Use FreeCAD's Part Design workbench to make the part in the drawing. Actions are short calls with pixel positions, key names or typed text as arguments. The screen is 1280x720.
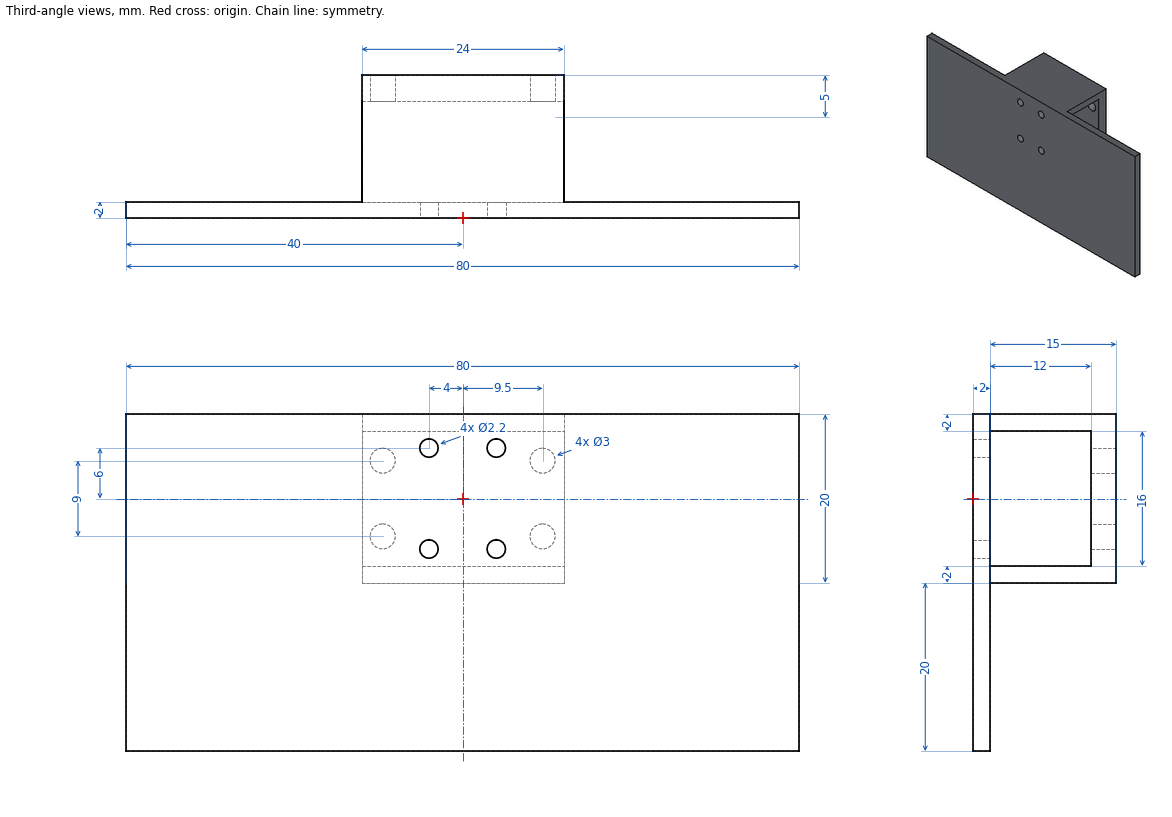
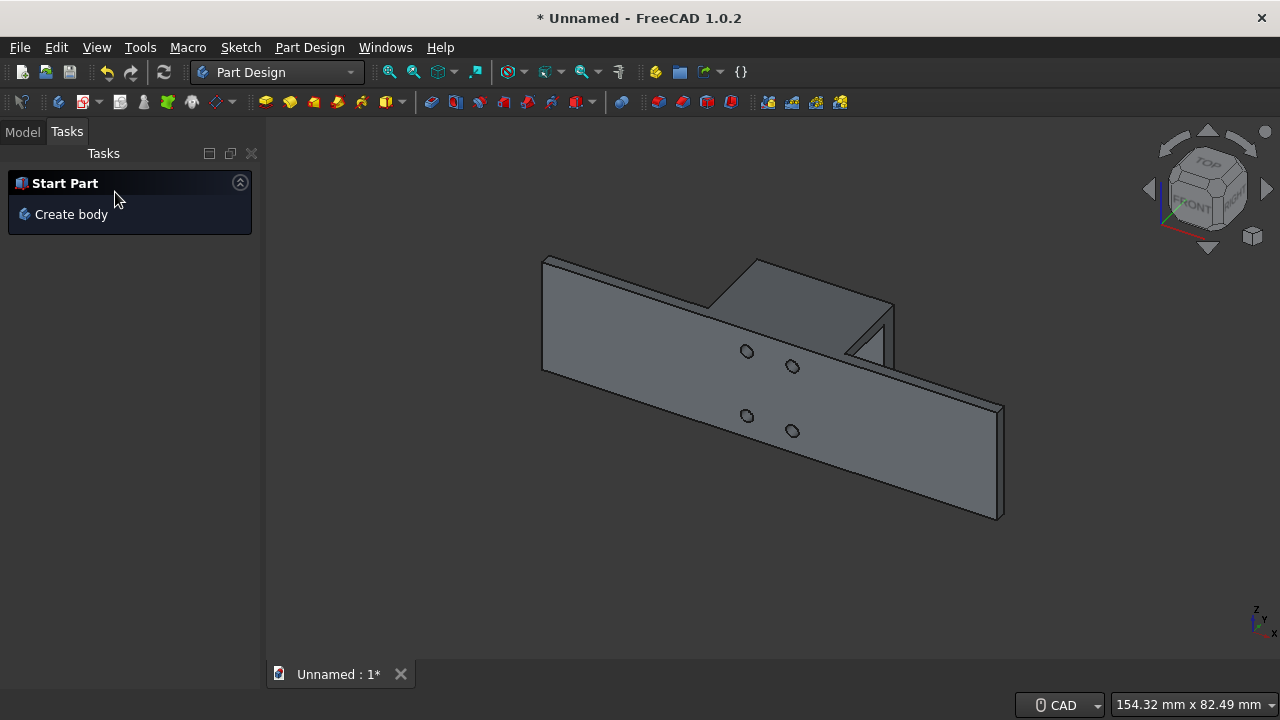
key(4)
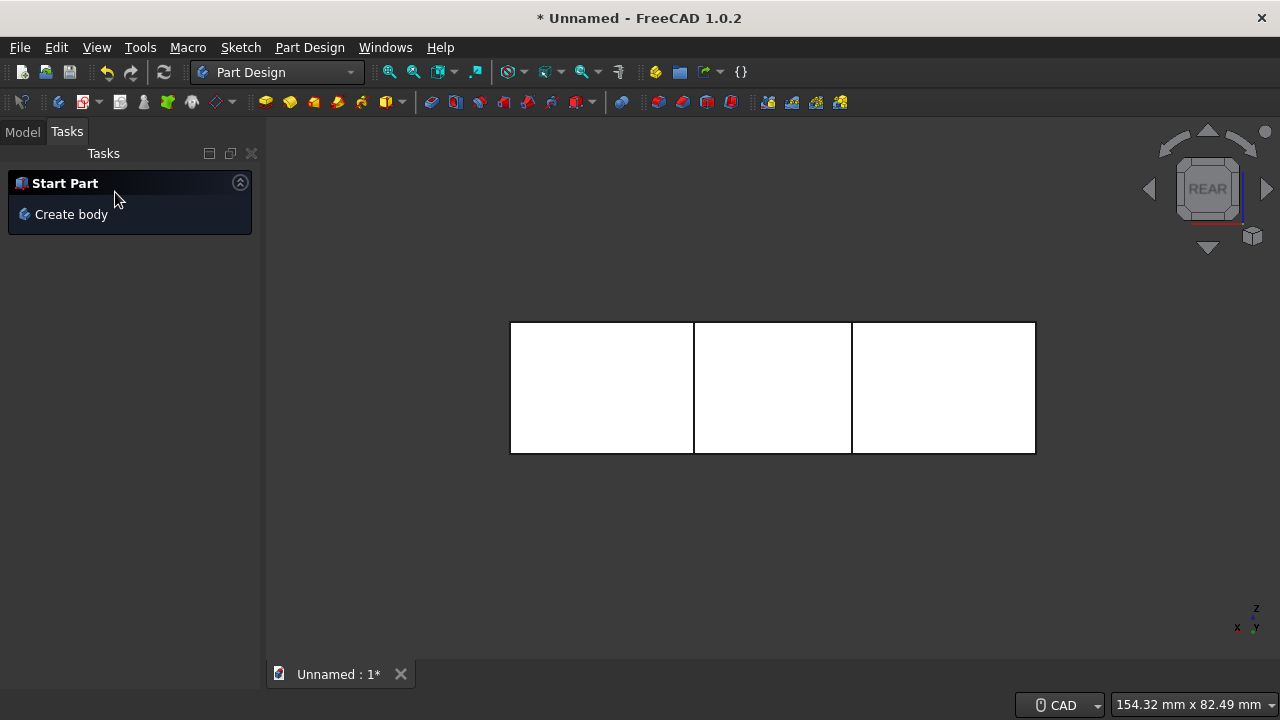
click(773, 387)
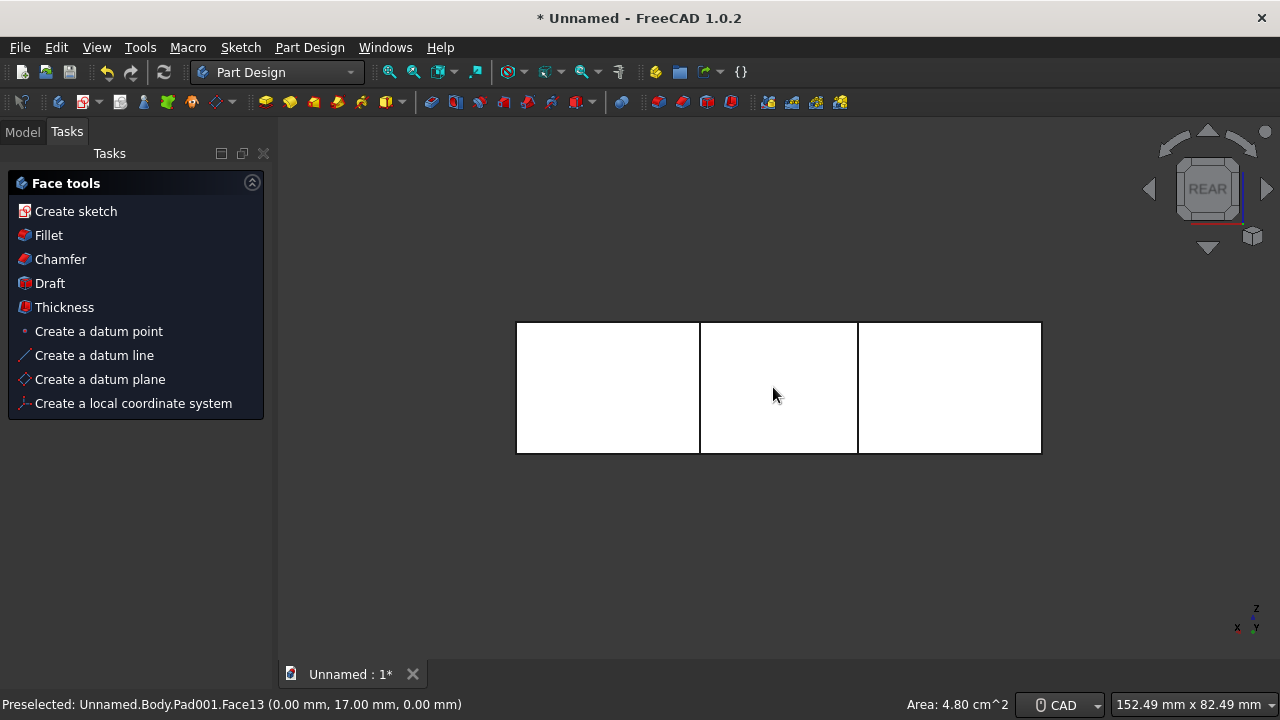
click(84, 102)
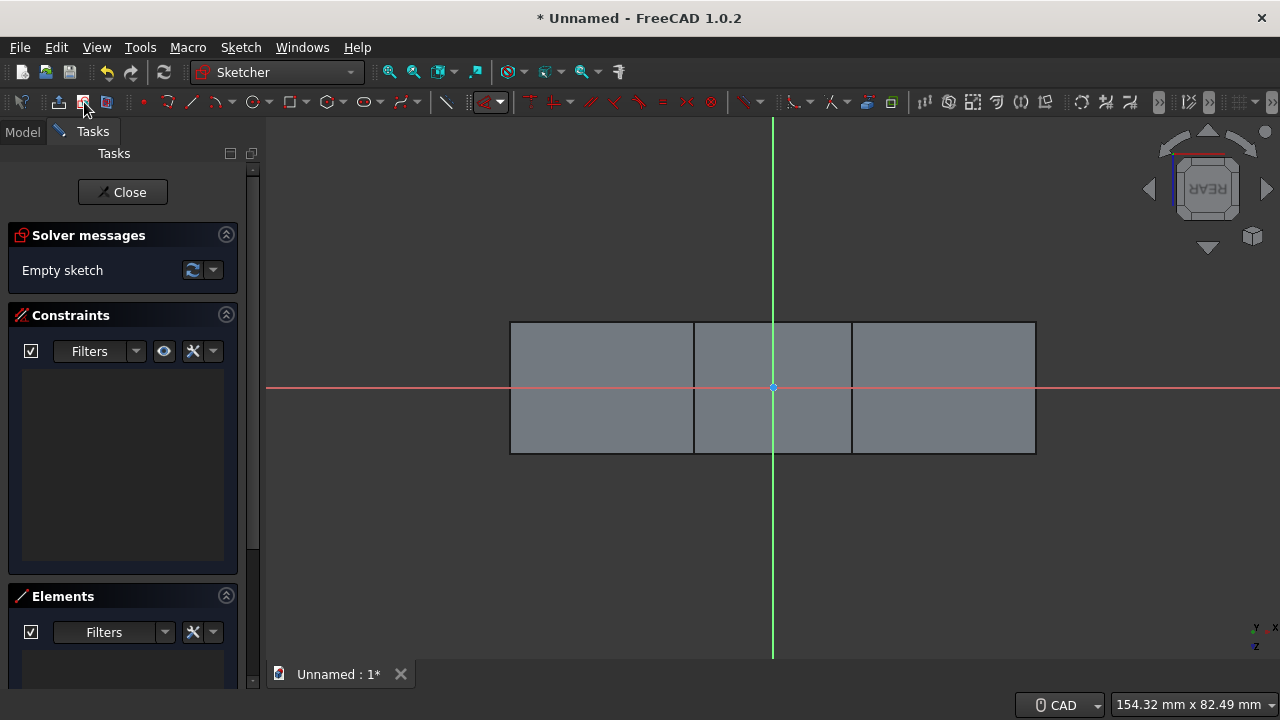
scroll(795, 388, up, 7)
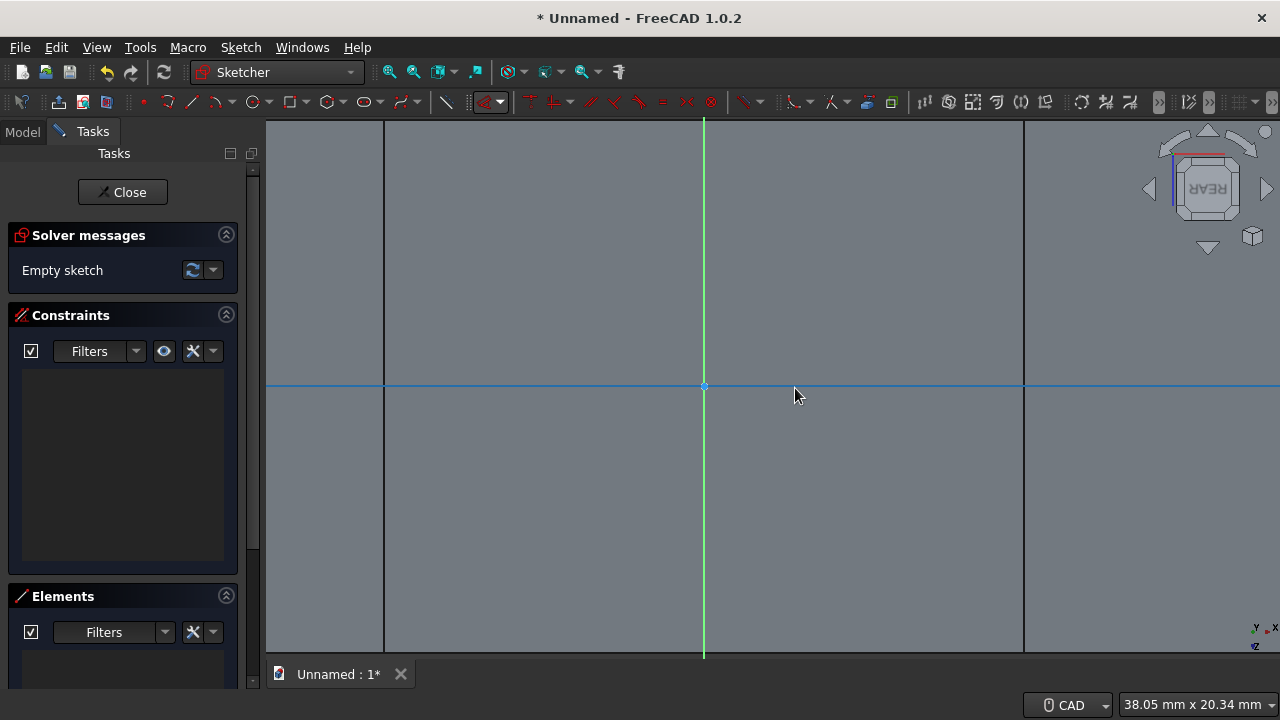
click(254, 102)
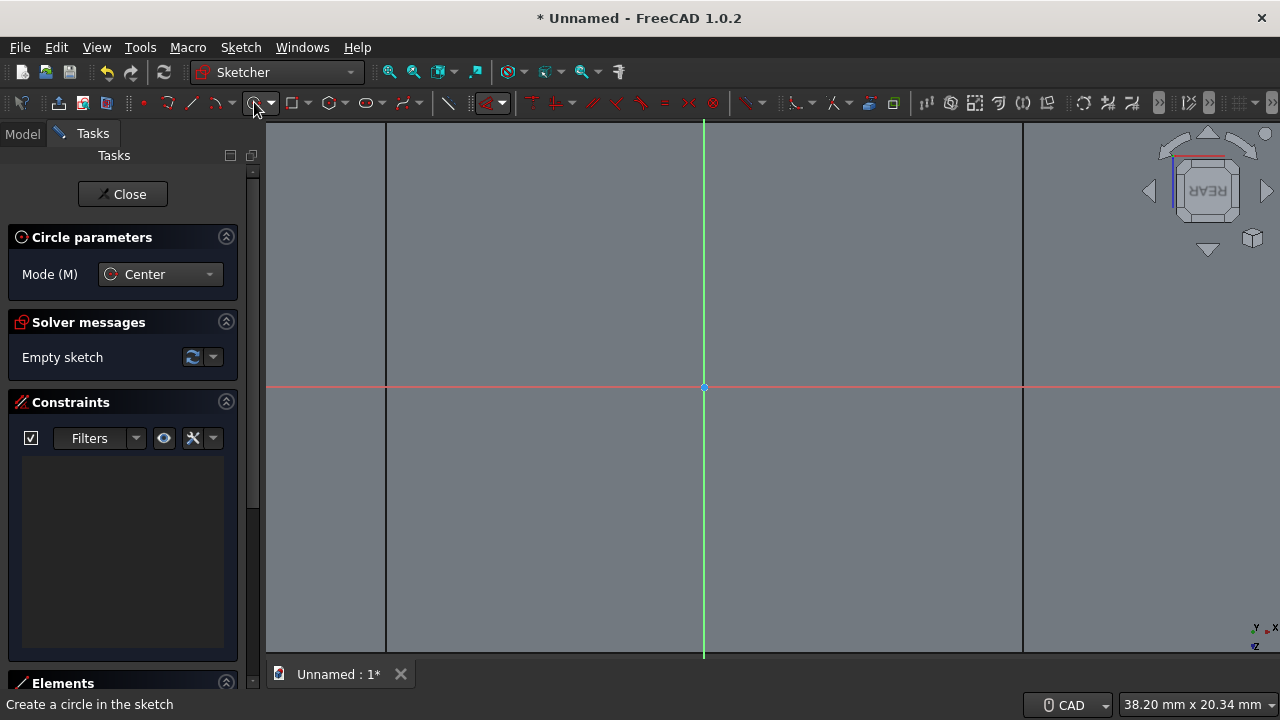
click(957, 507)
click(985, 479)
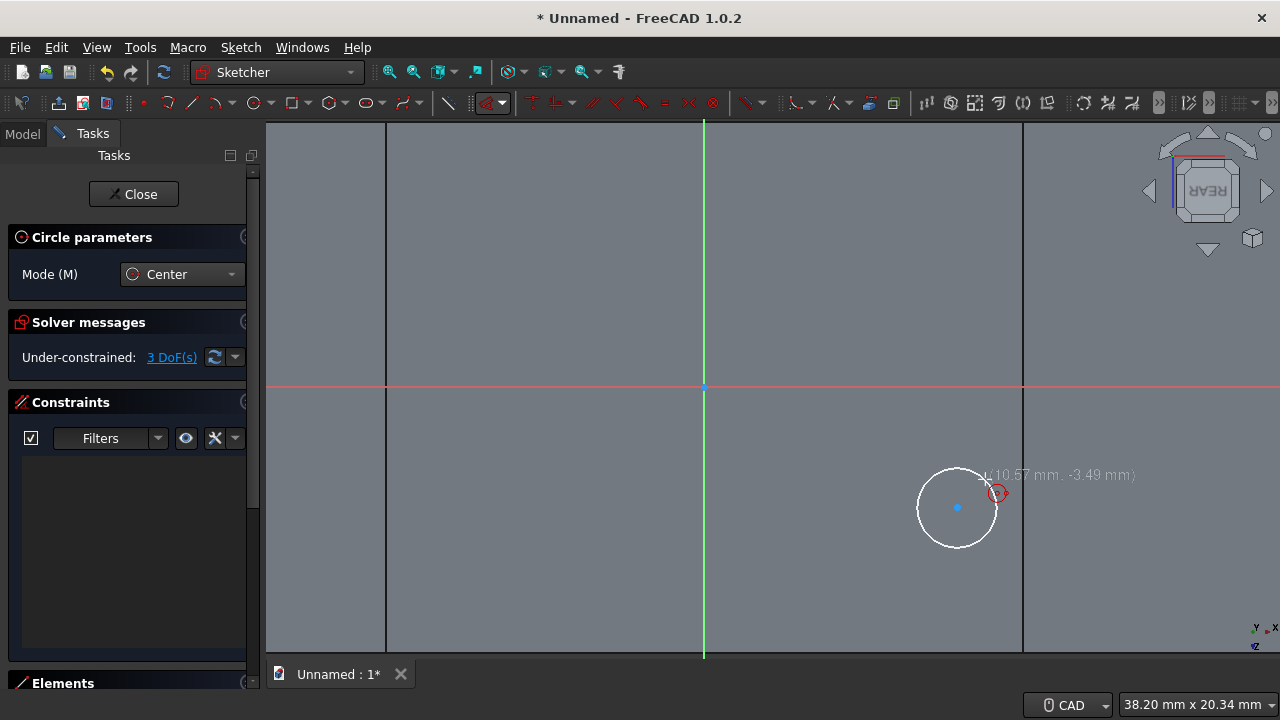
click(452, 507)
click(480, 479)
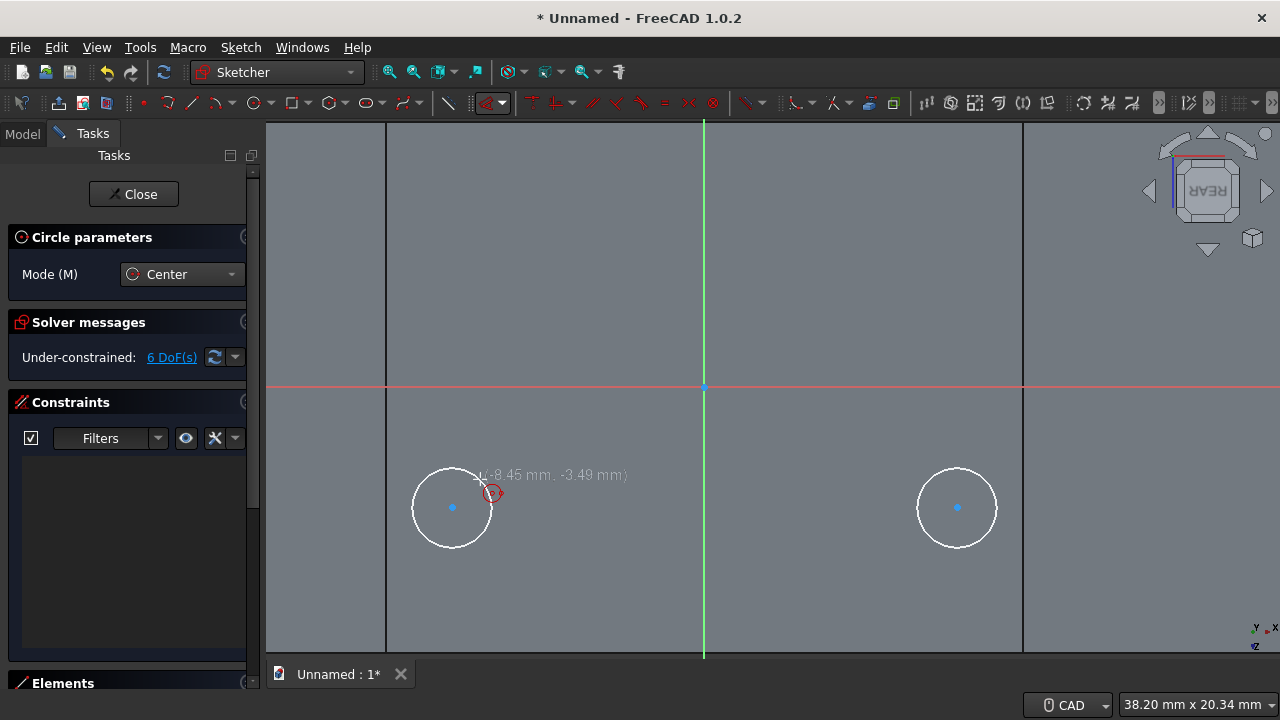
click(452, 268)
click(480, 240)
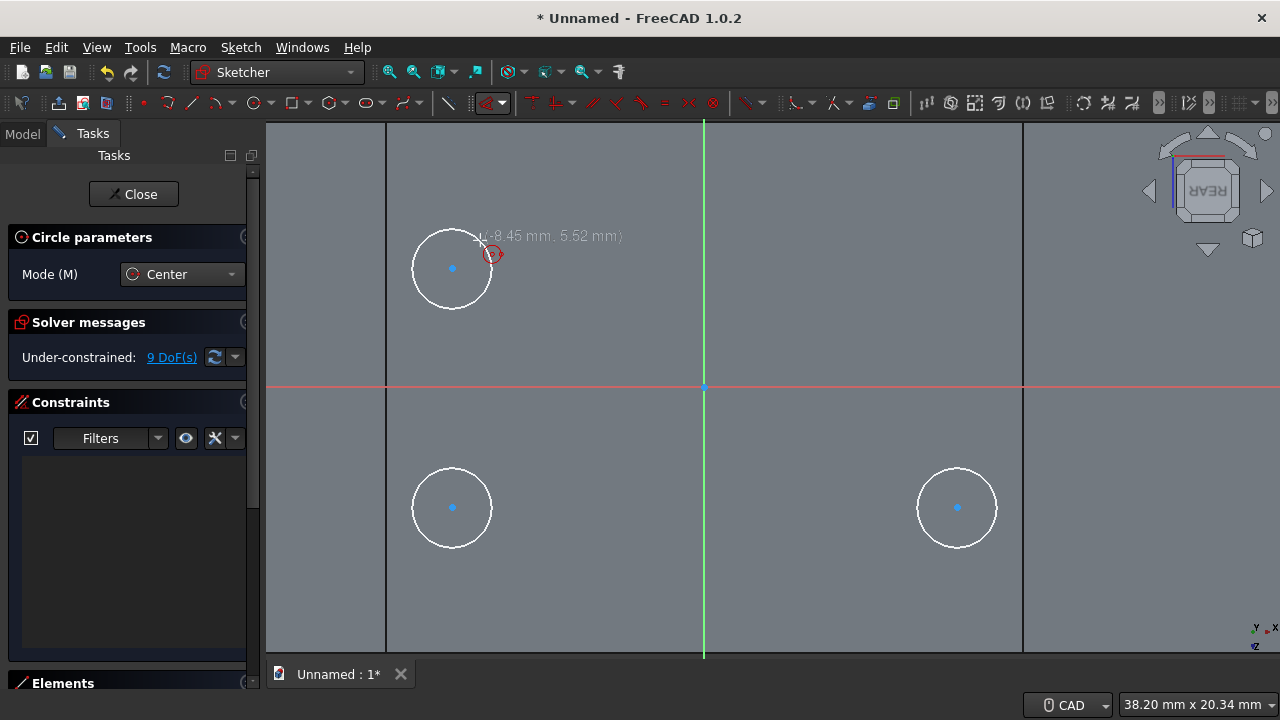
click(957, 268)
click(985, 240)
key(Escape)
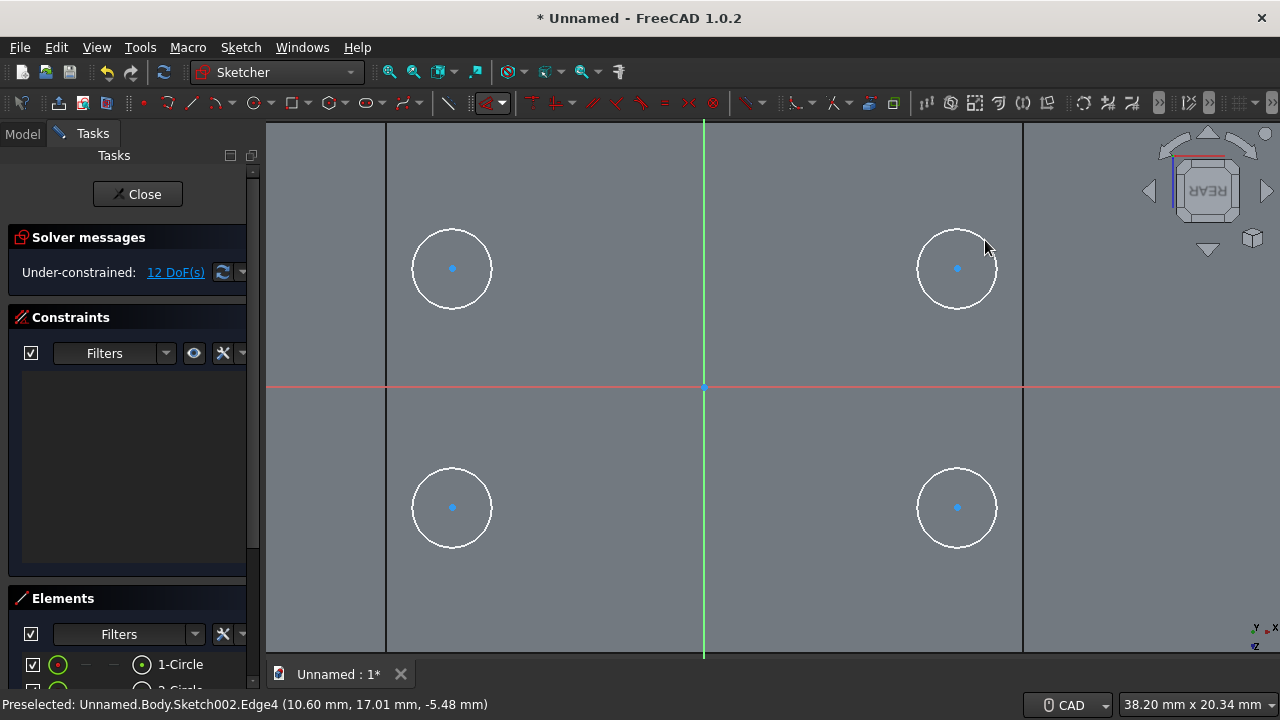
click(985, 480)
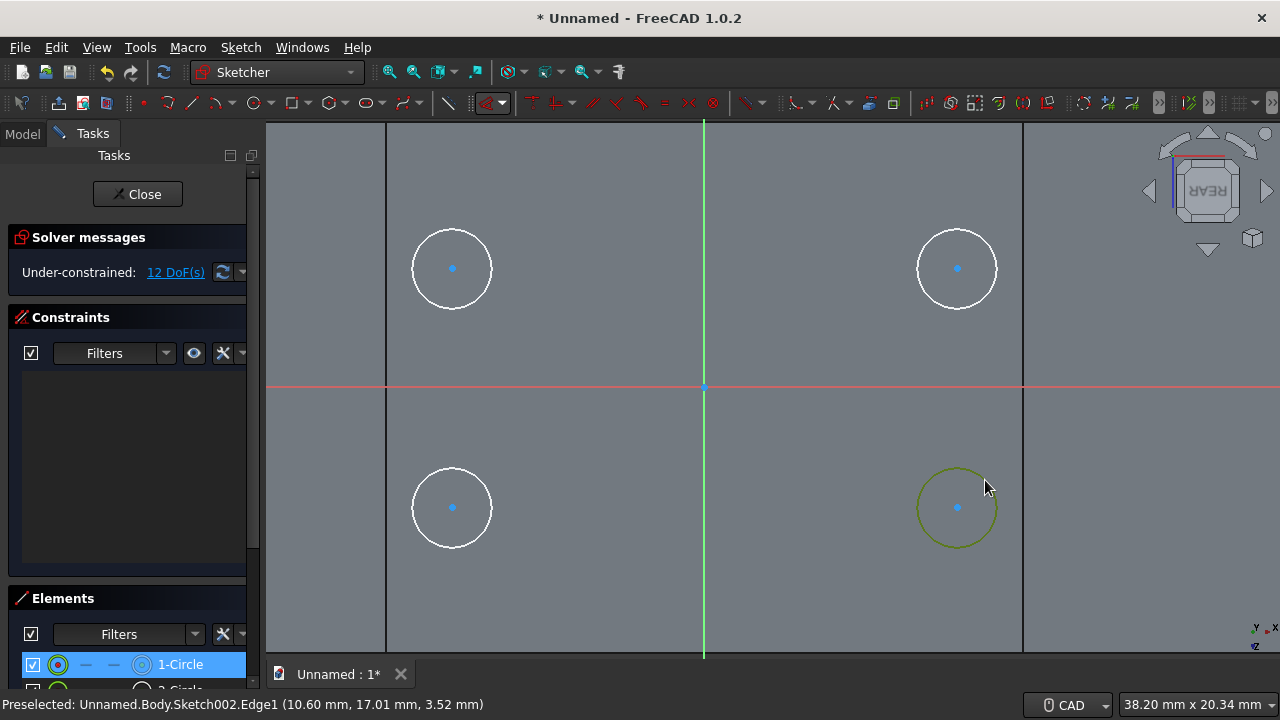
click(480, 480)